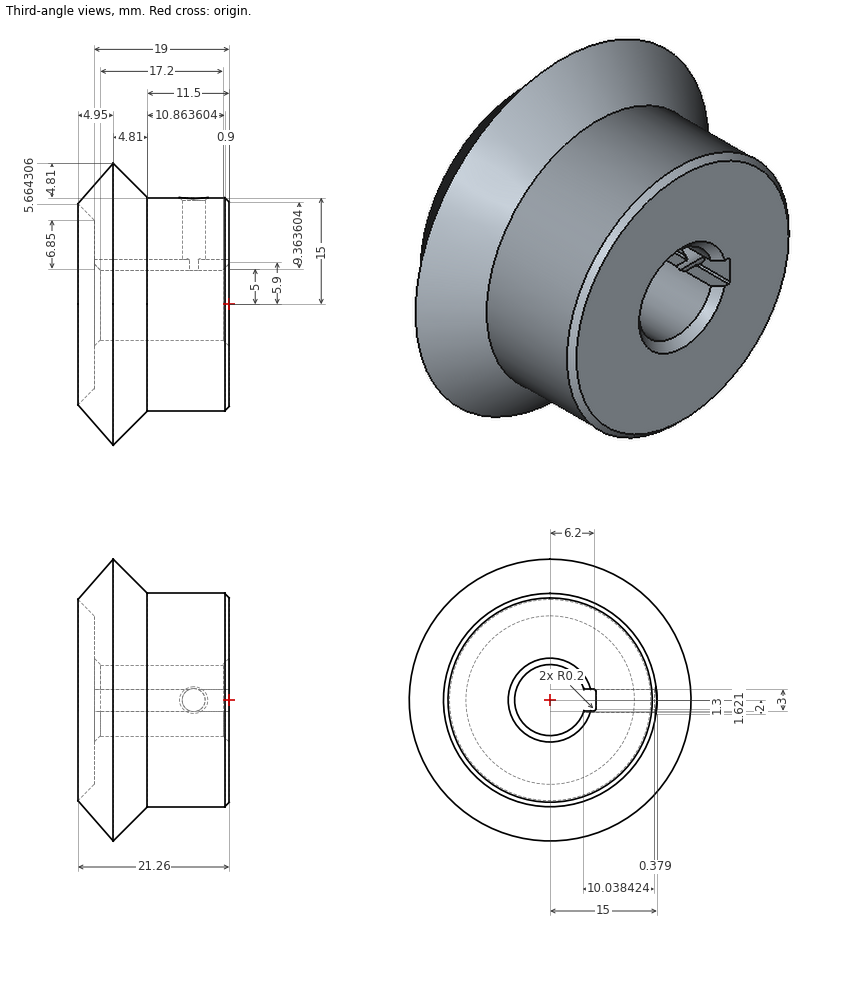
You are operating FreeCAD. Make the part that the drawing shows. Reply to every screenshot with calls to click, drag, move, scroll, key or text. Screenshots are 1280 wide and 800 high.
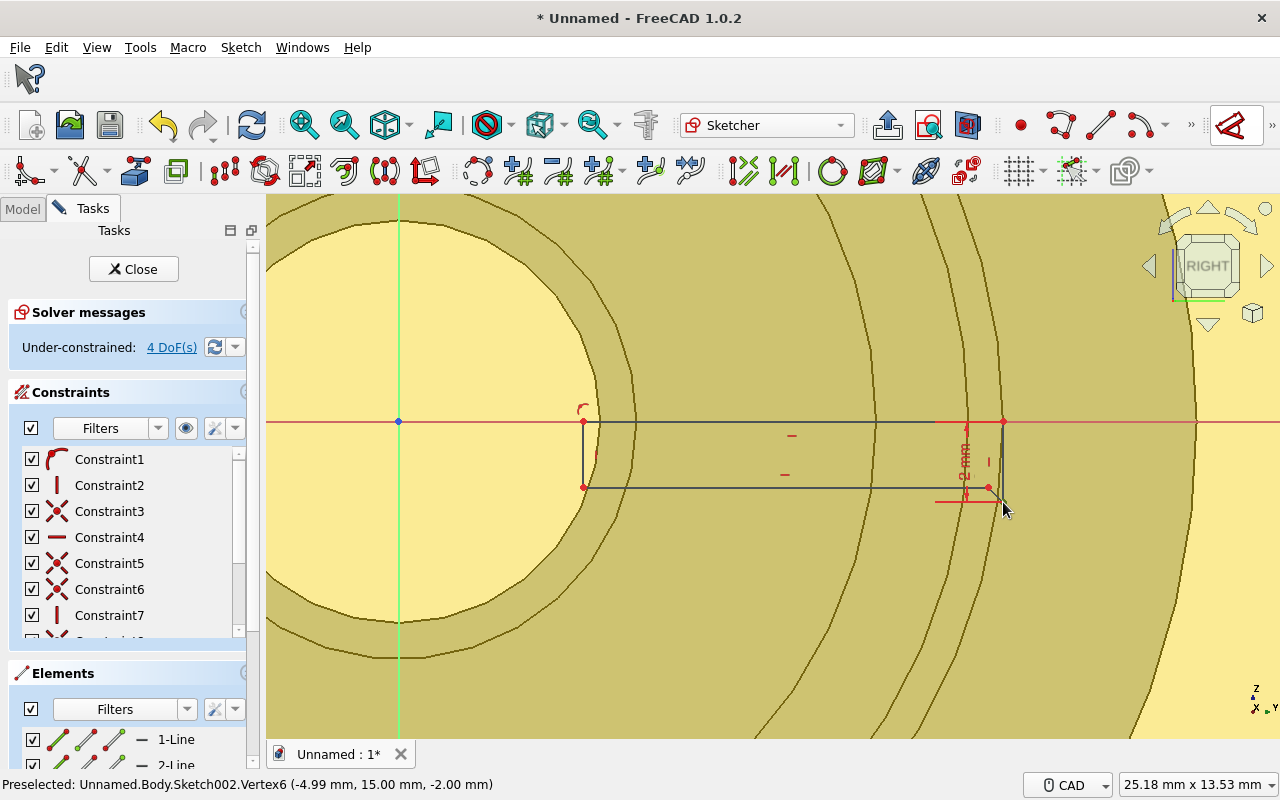
click(1258, 126)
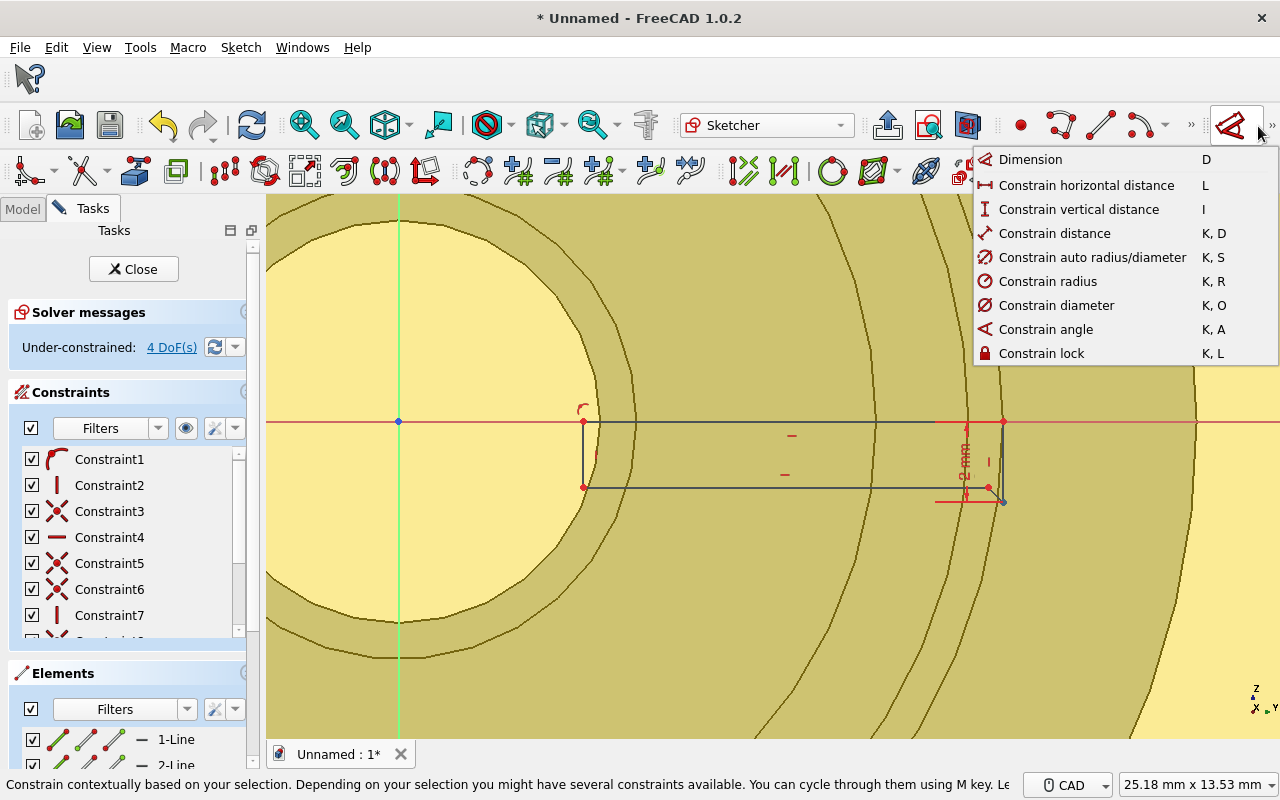
click(1126, 185)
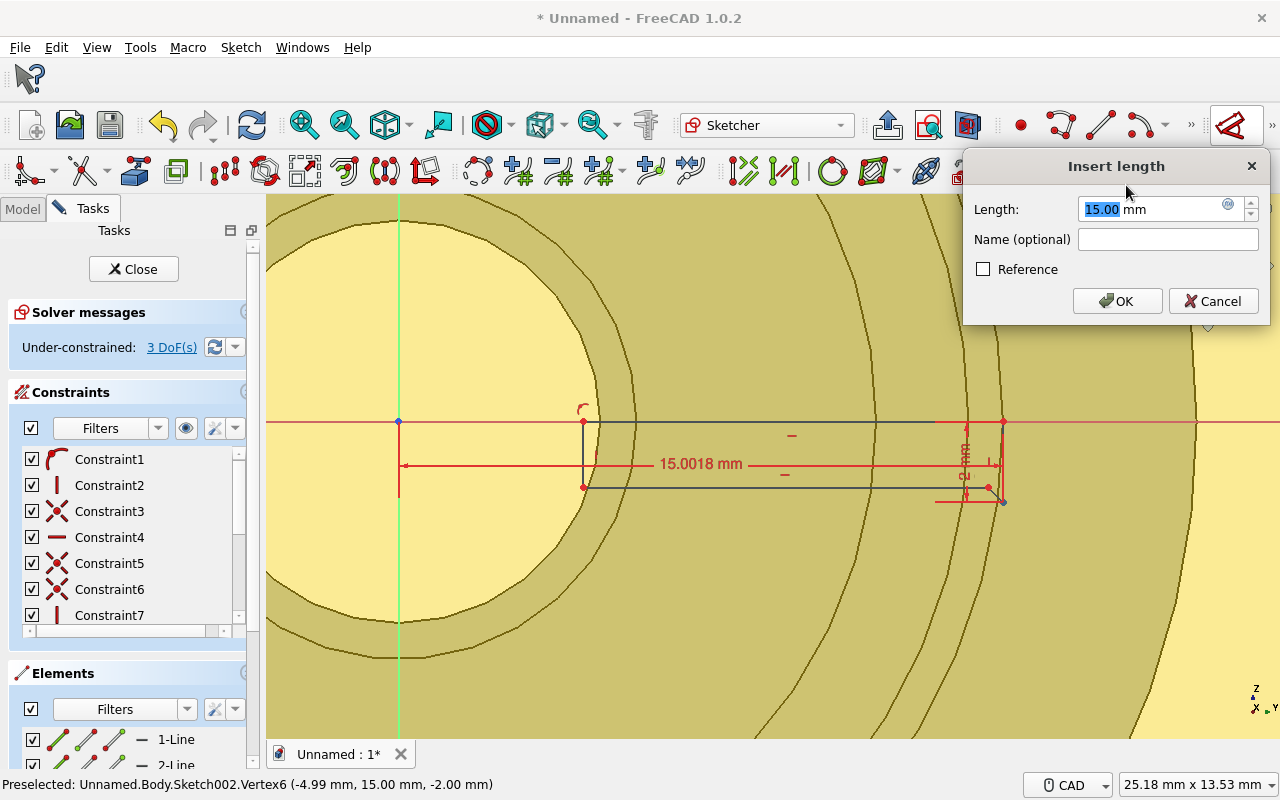
text(15)
key(Return)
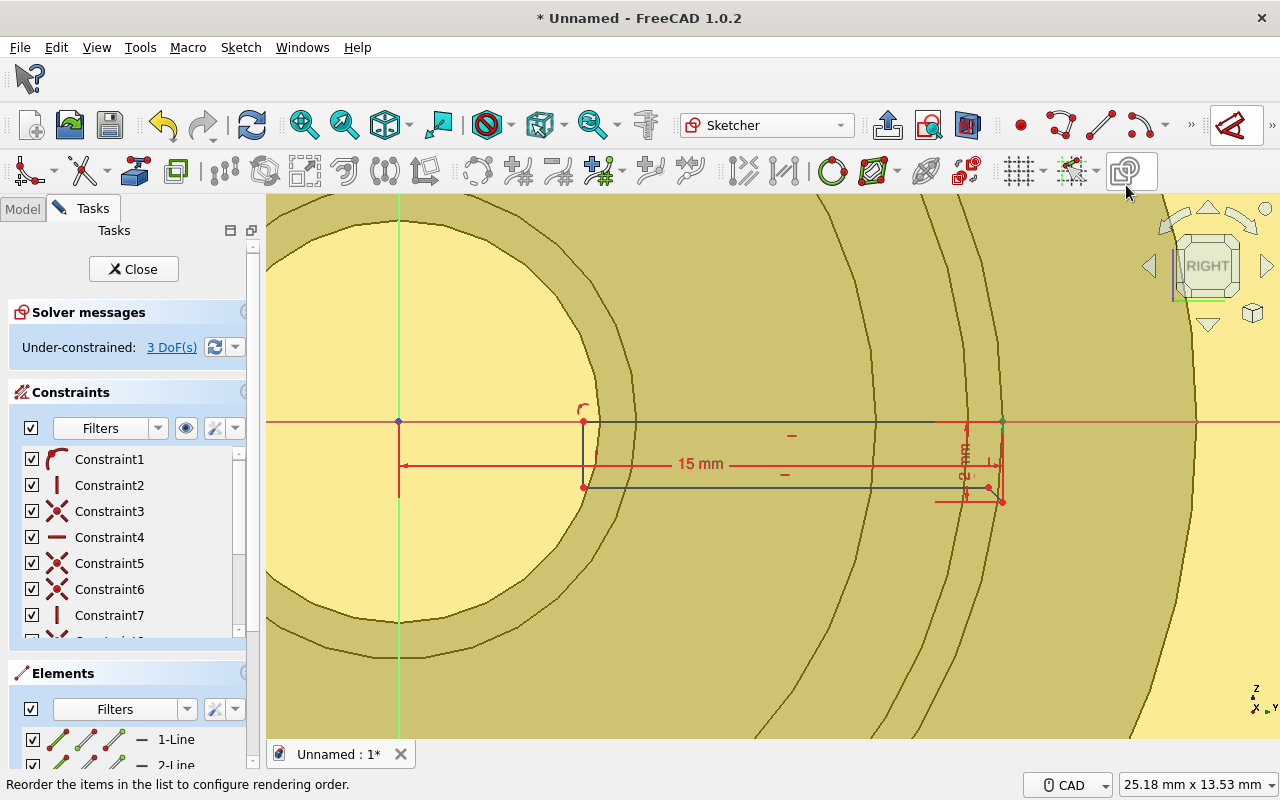
click(583, 442)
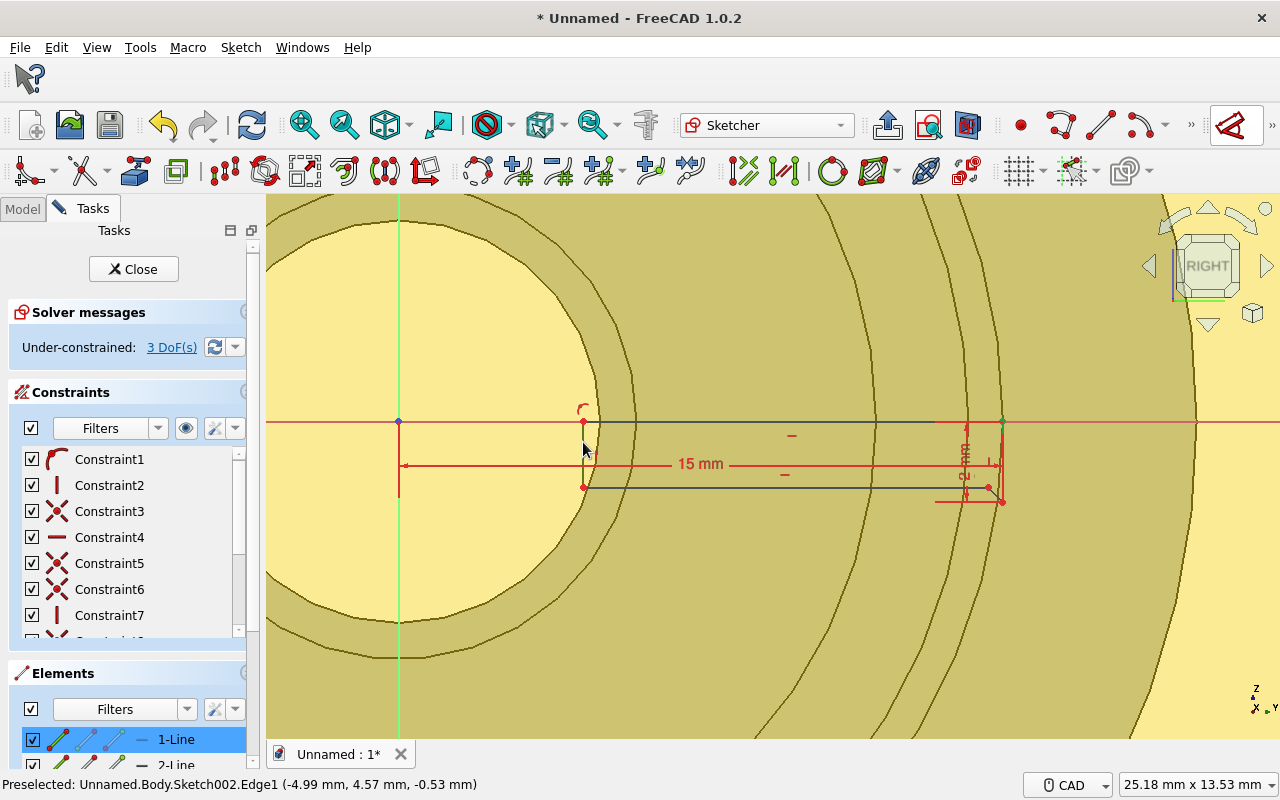
click(1258, 126)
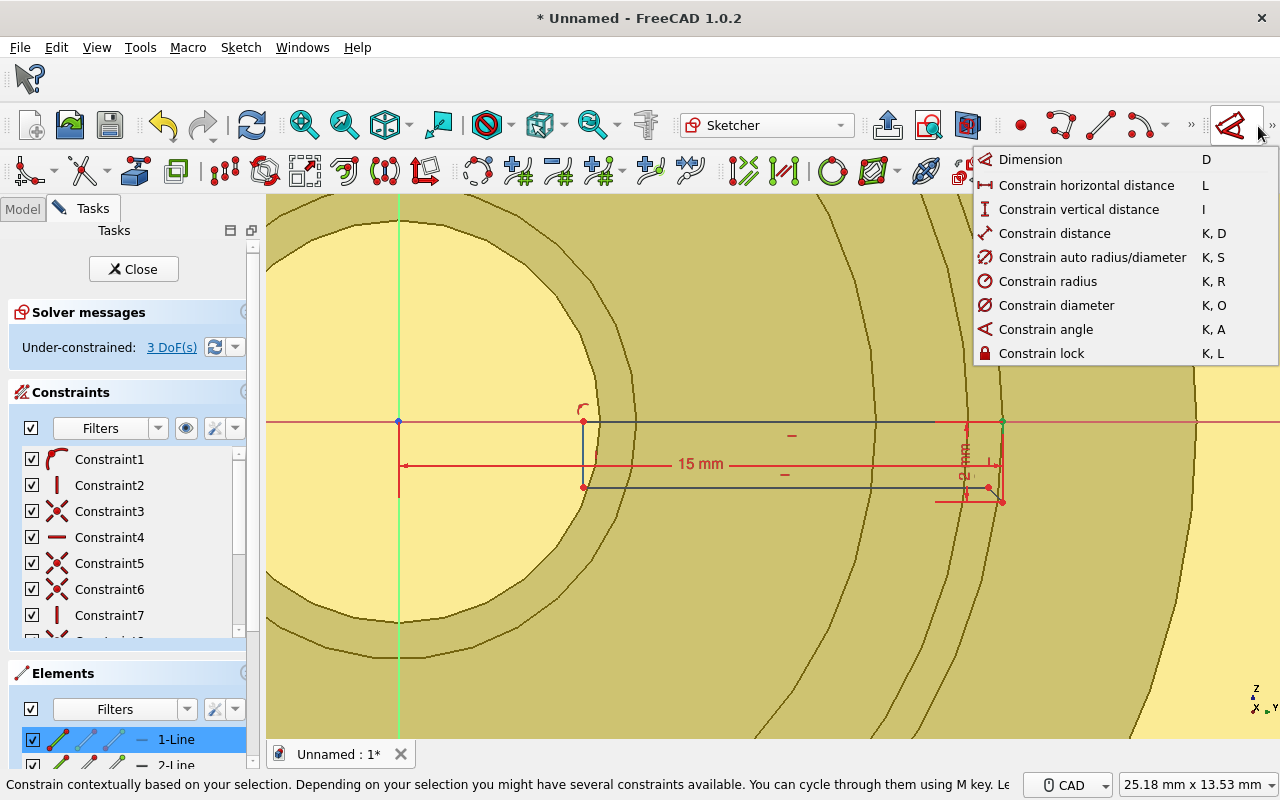
click(1126, 209)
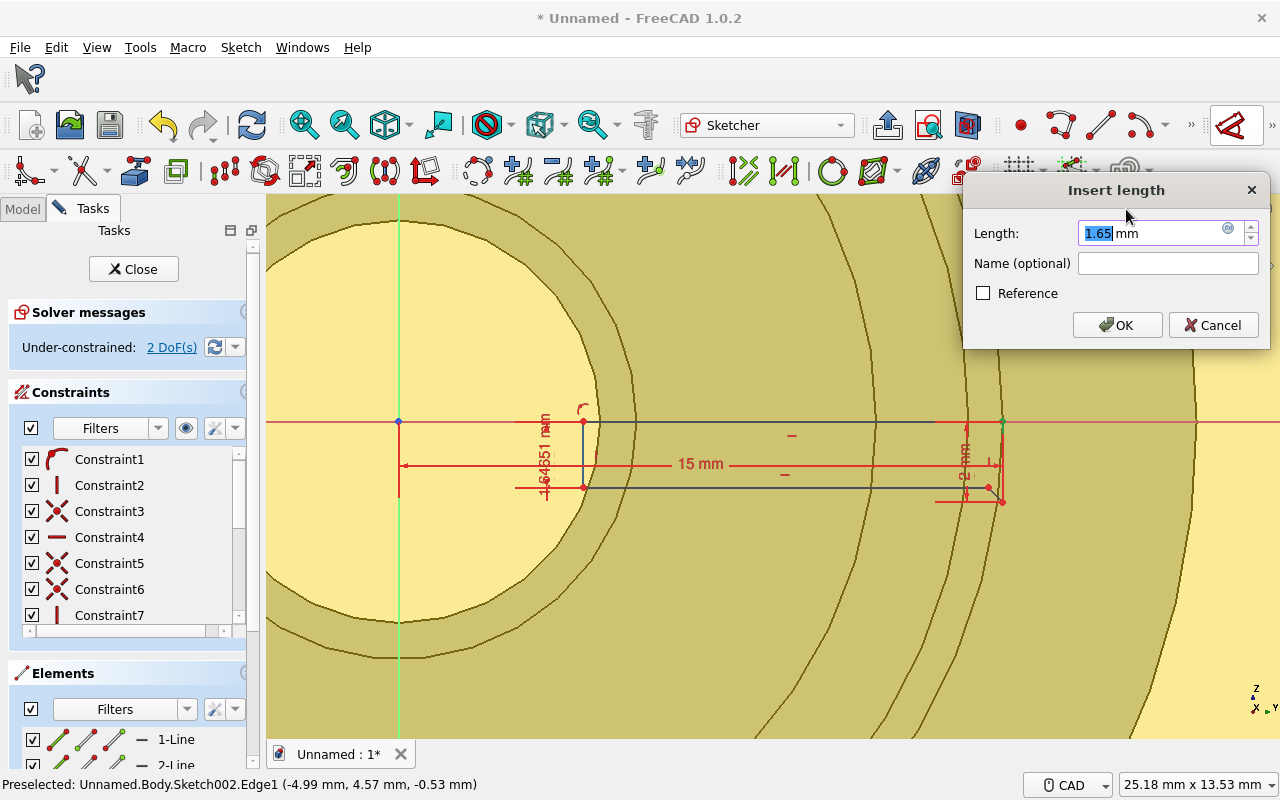
text(1.621)
key(Return)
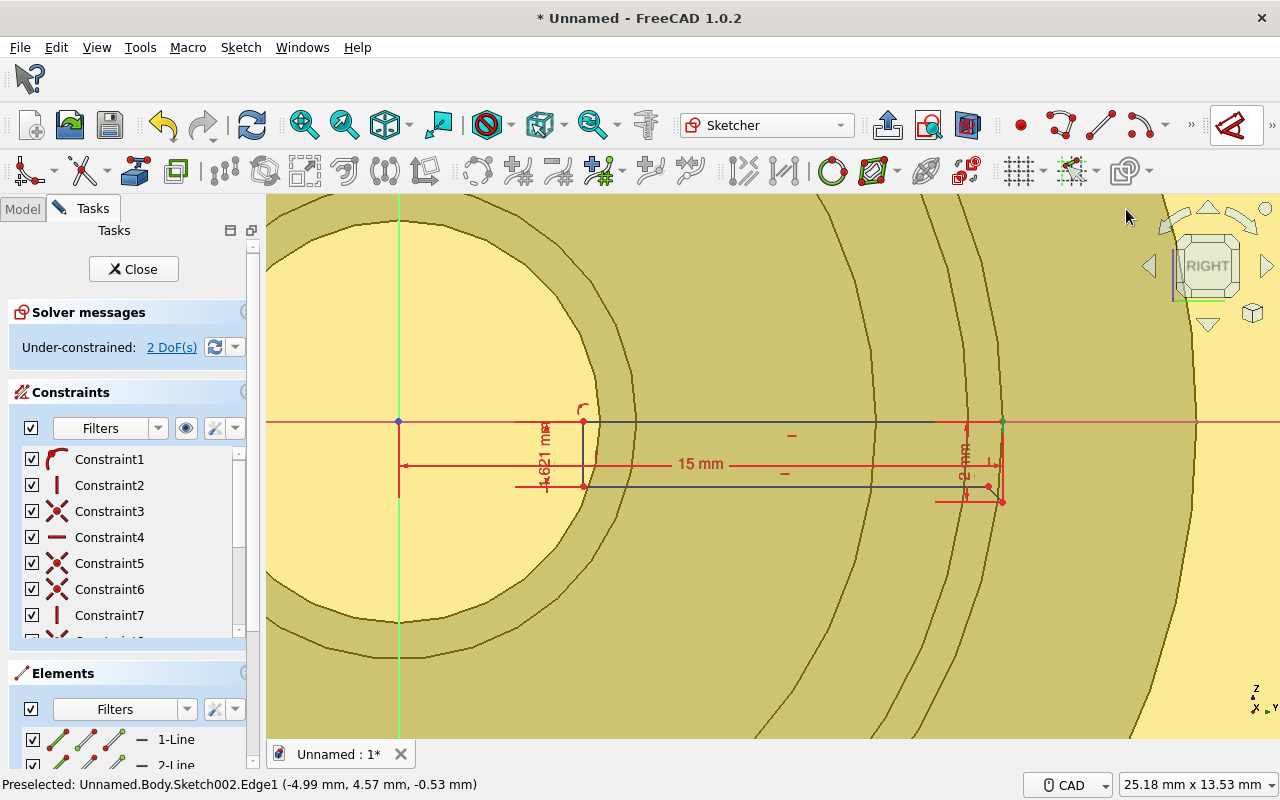
scroll(994, 493, up, 5)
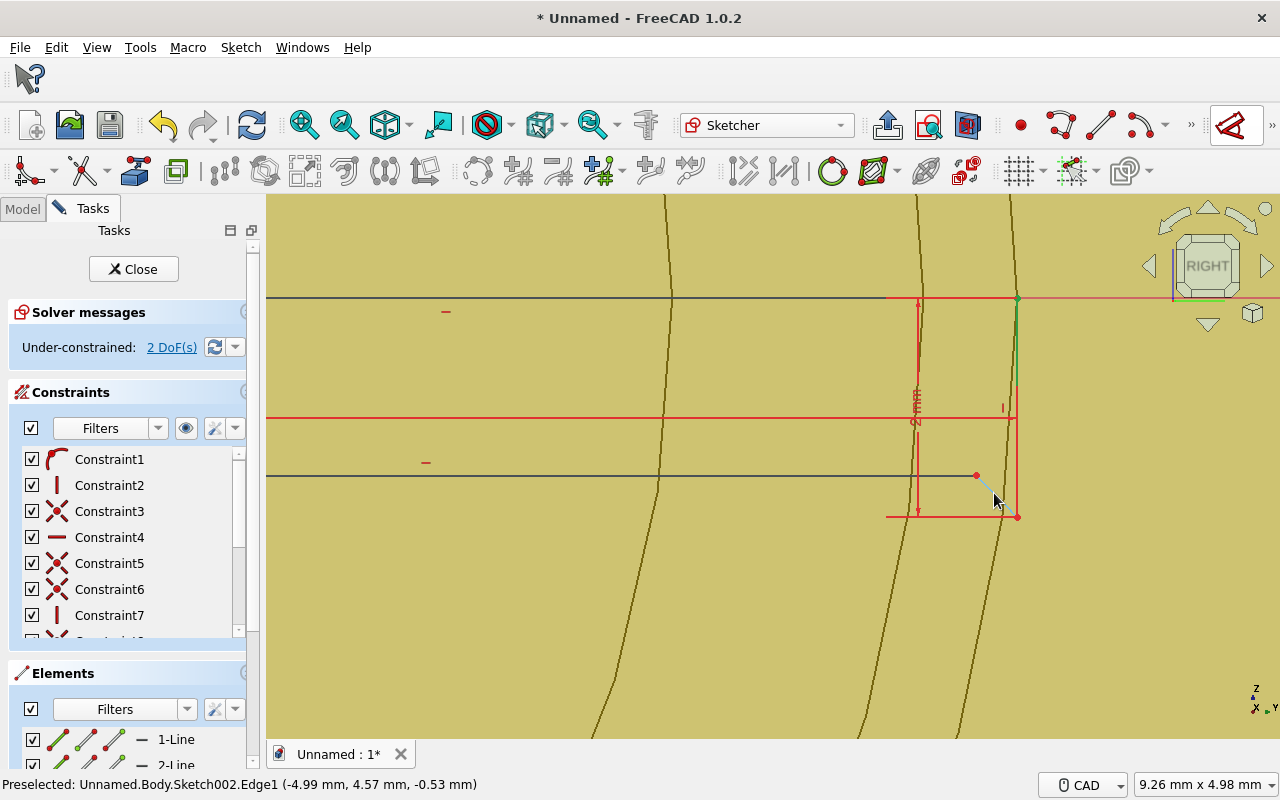
click(993, 492)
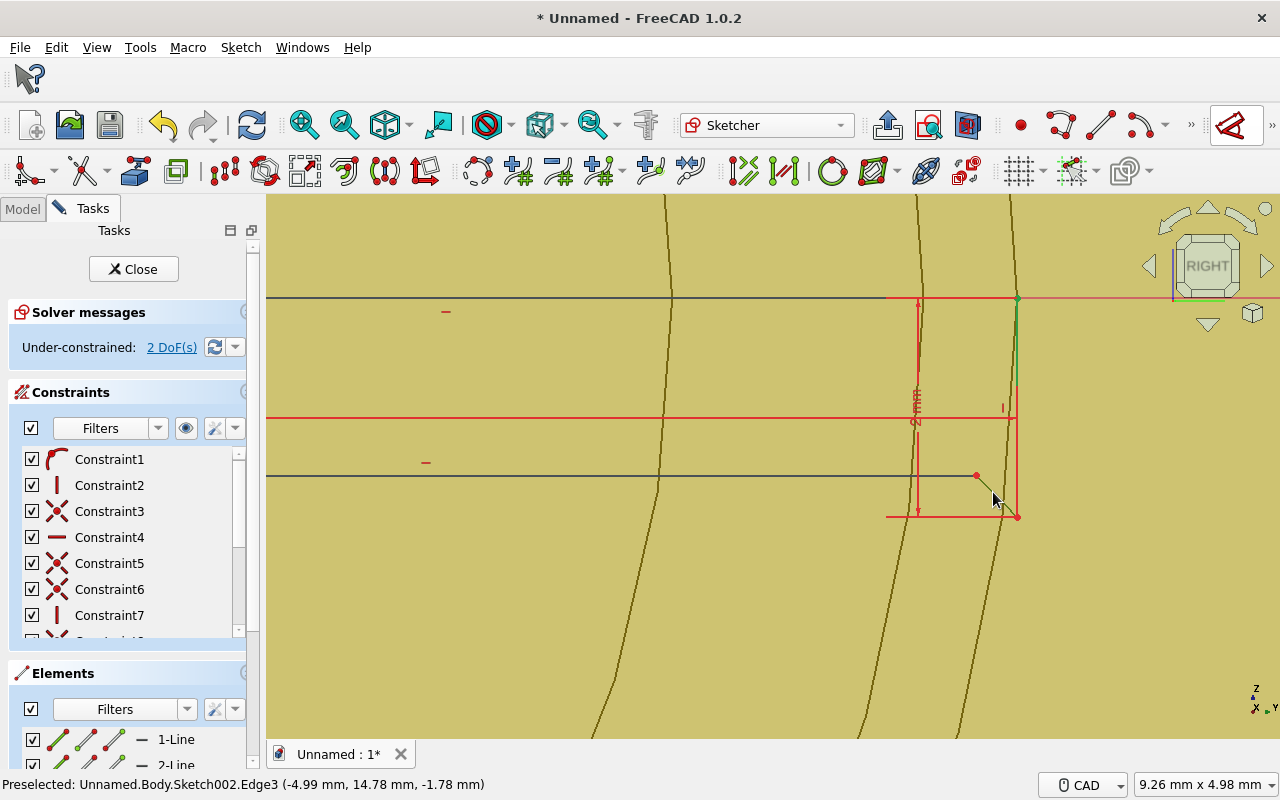
key(l)